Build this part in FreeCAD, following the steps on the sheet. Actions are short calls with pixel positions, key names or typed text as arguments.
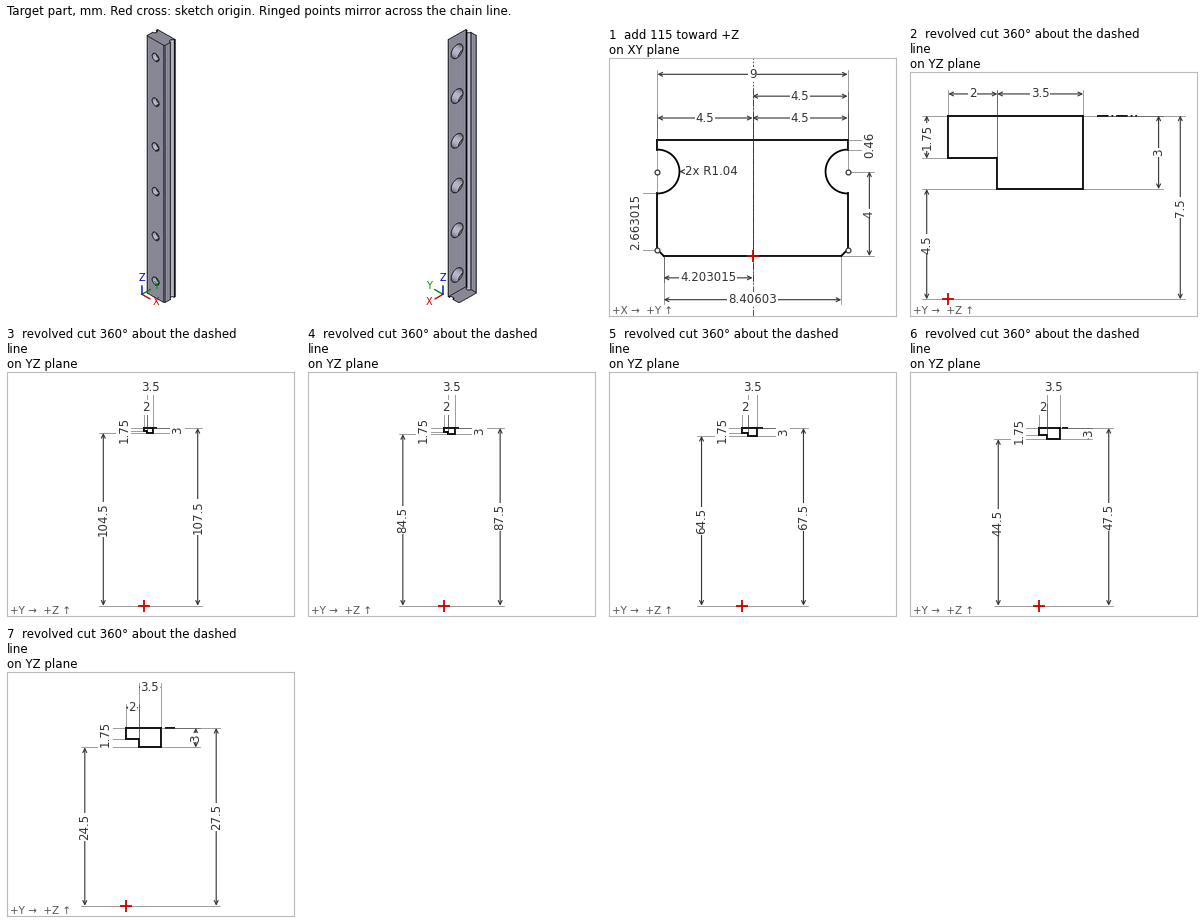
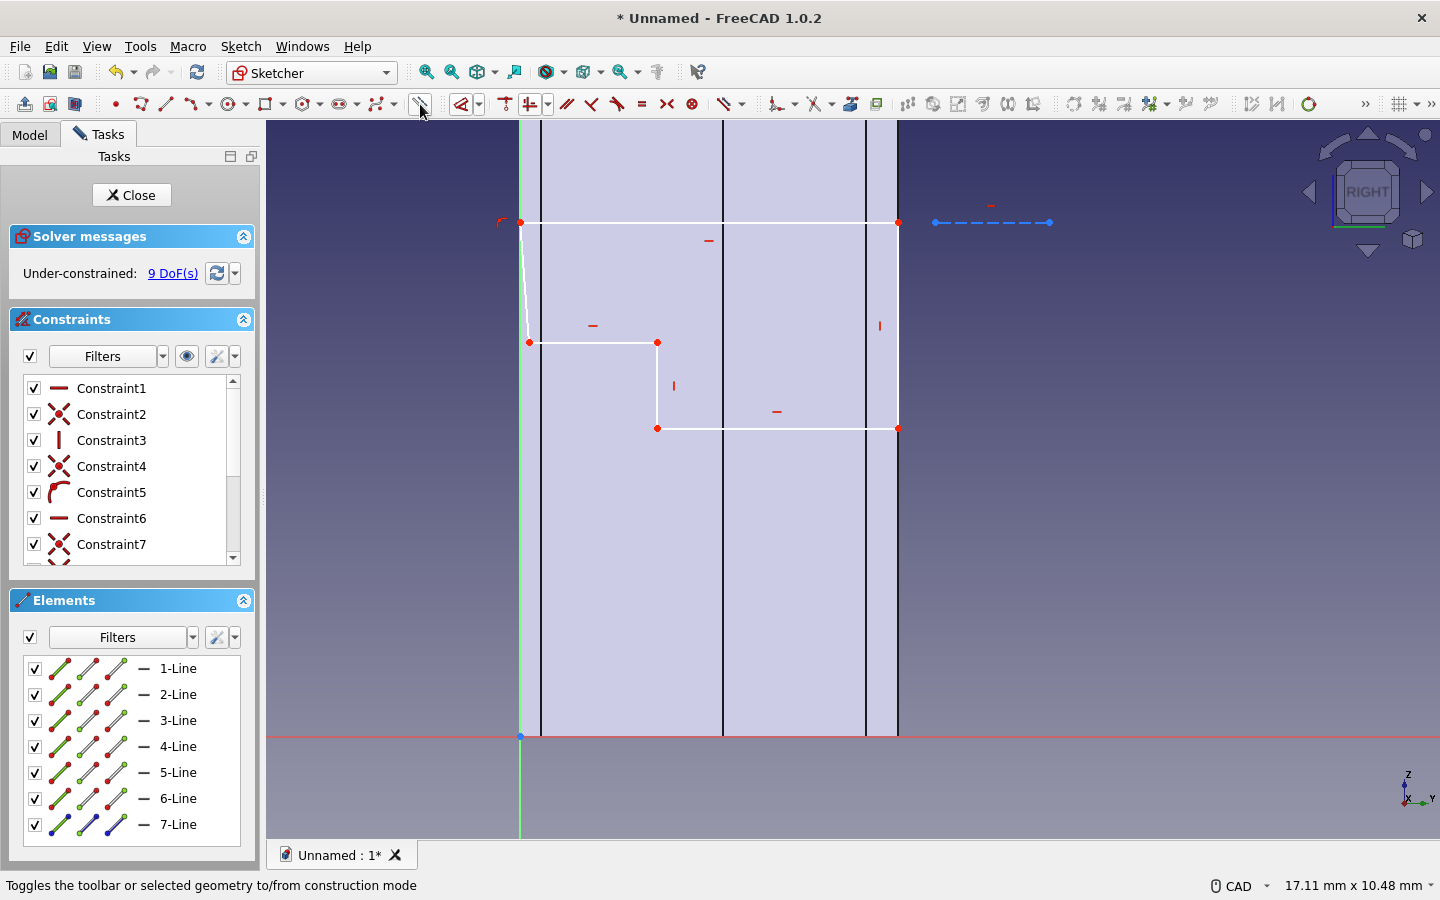
click(523, 259)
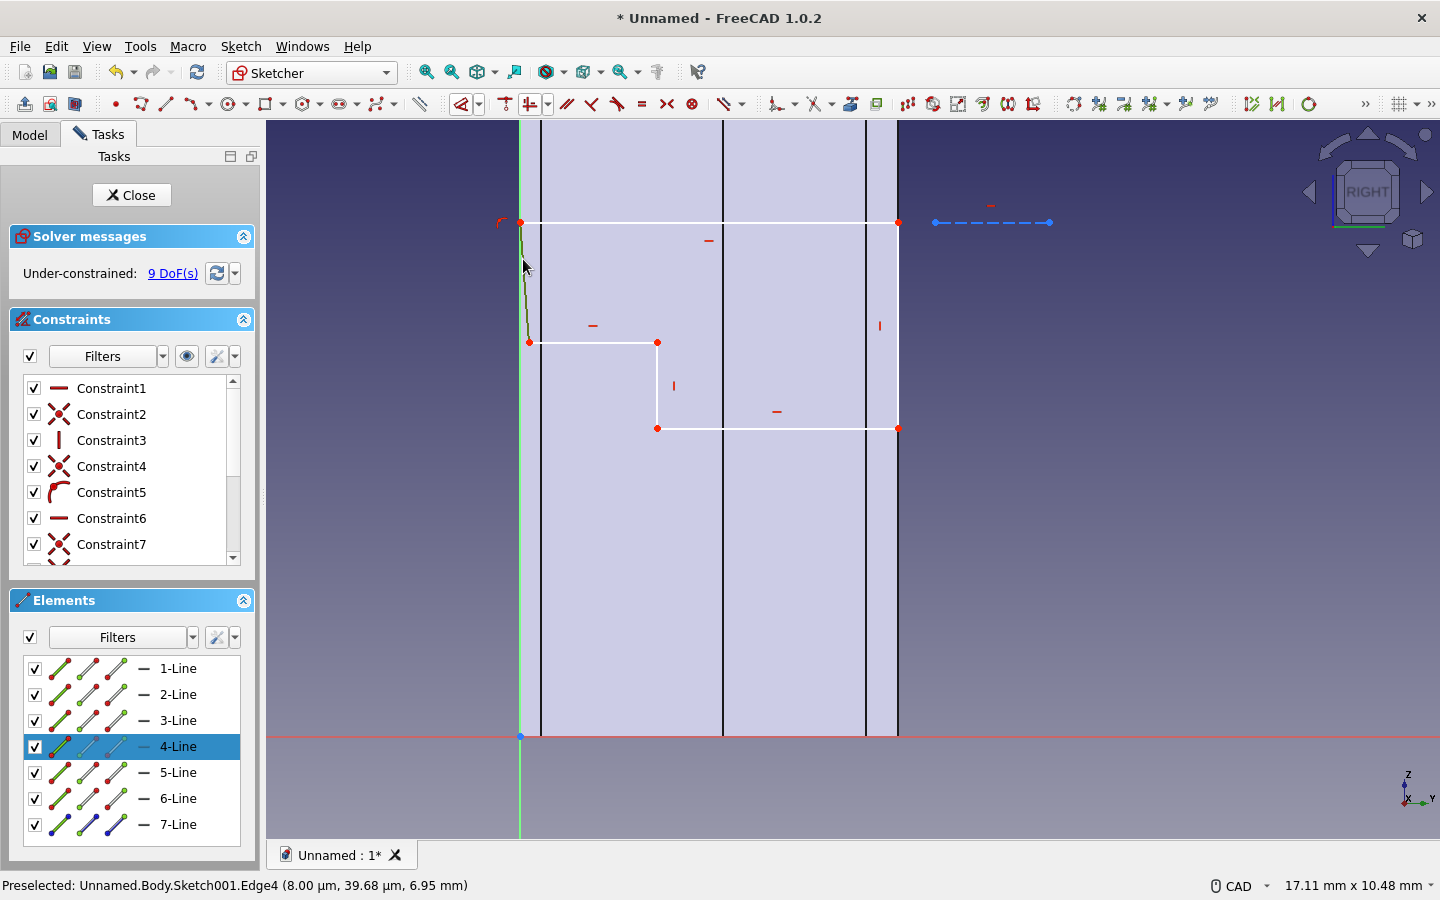
key(v)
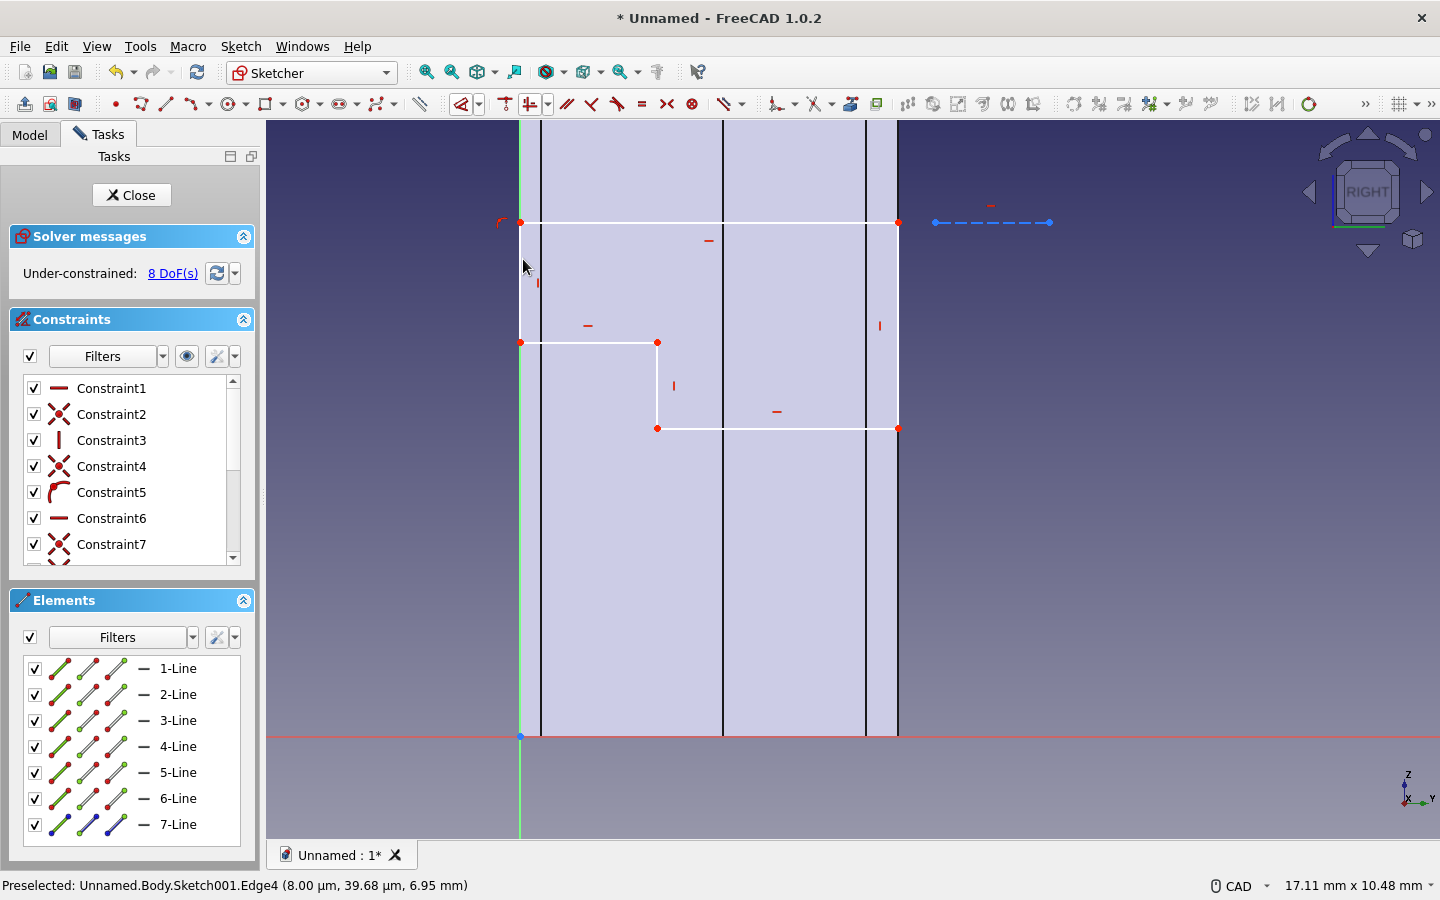
click(460, 104)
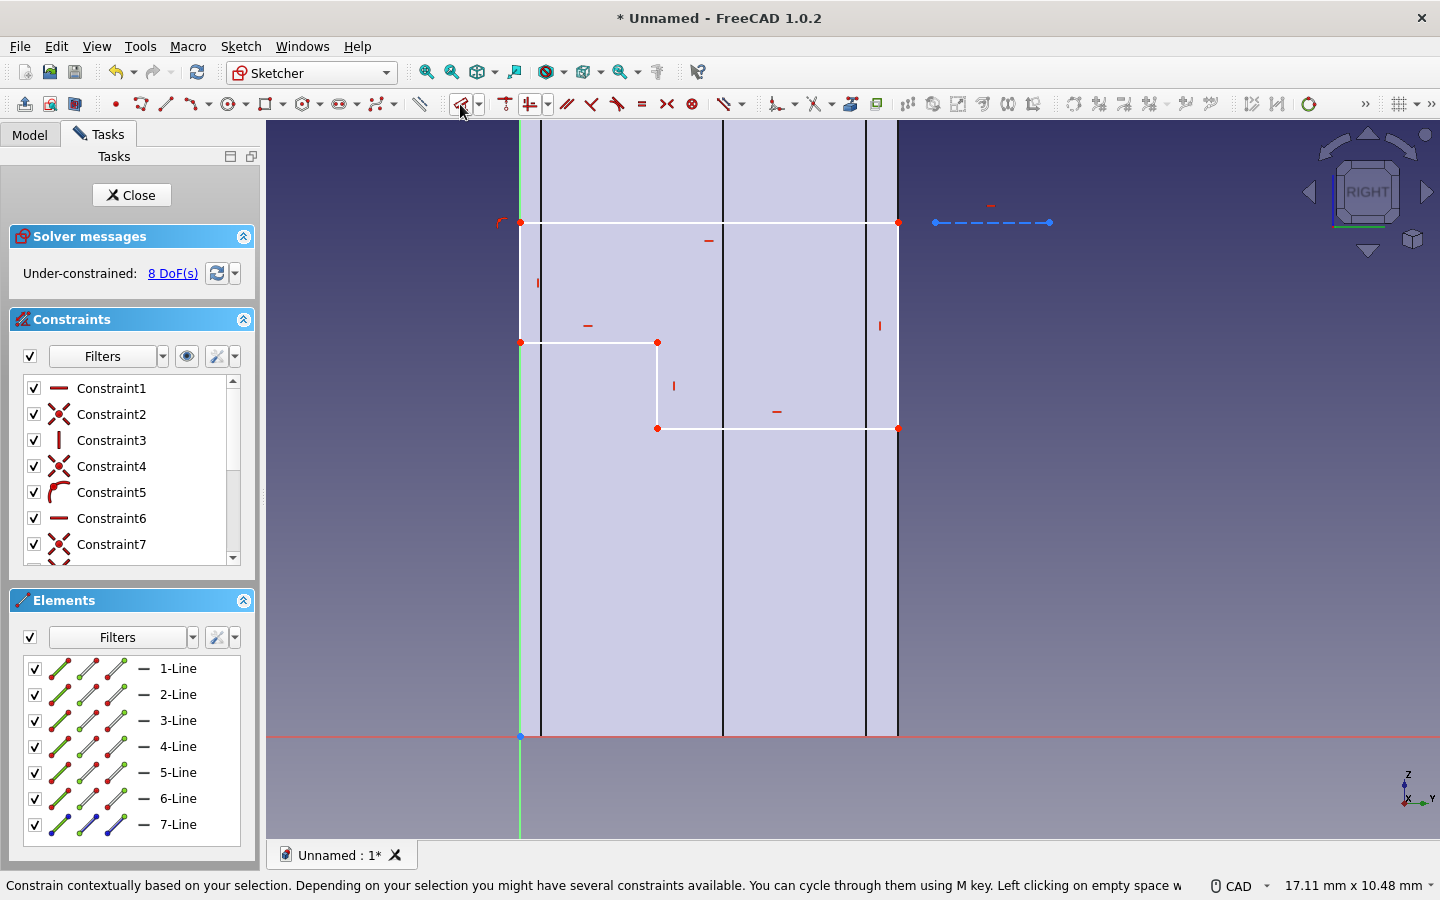
click(898, 367)
click(932, 326)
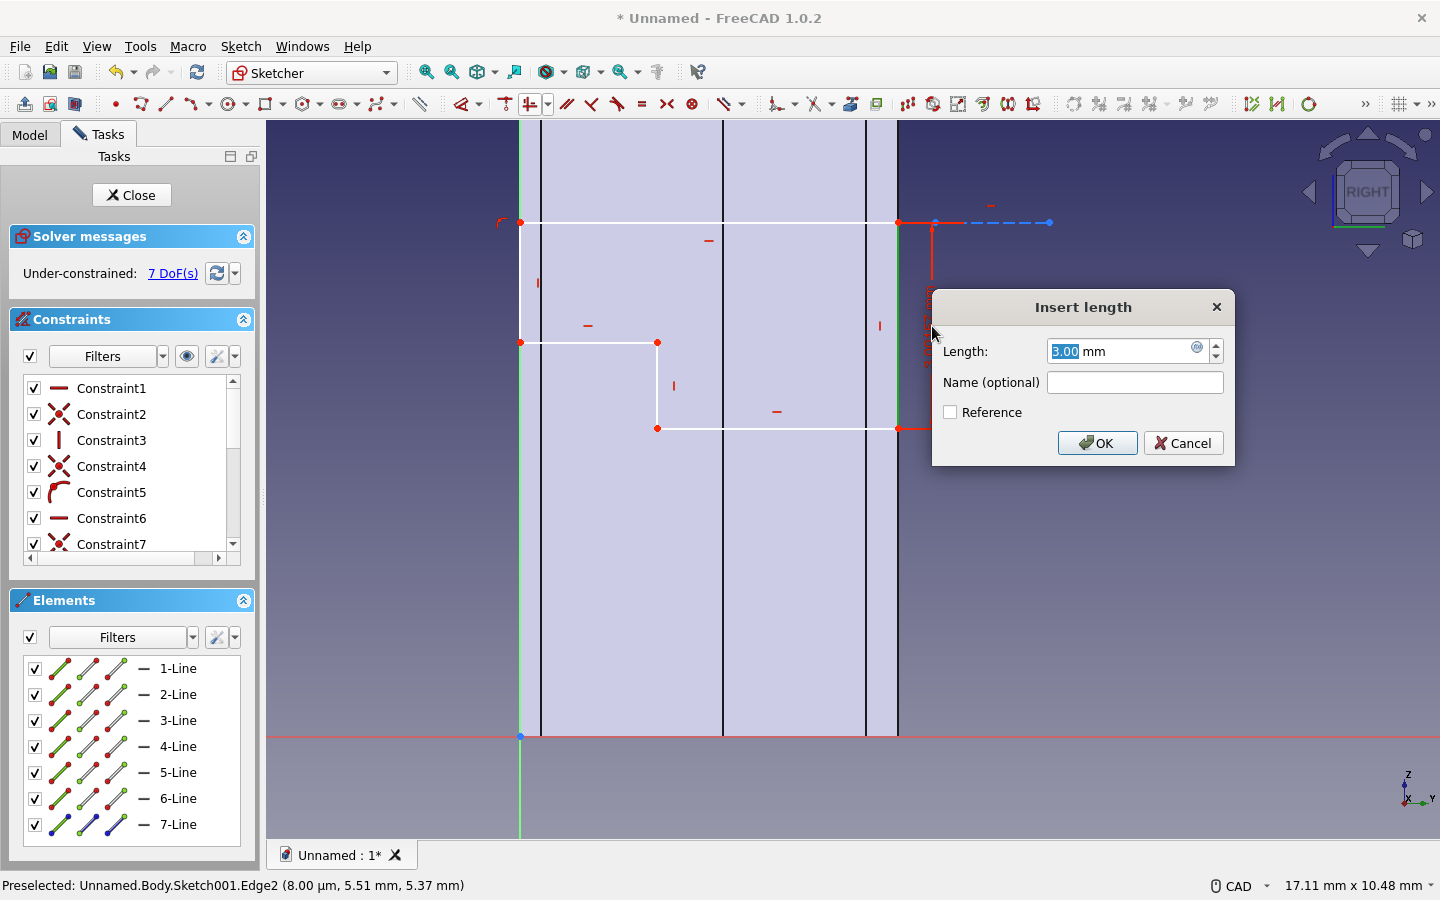
text(3)
key(Return)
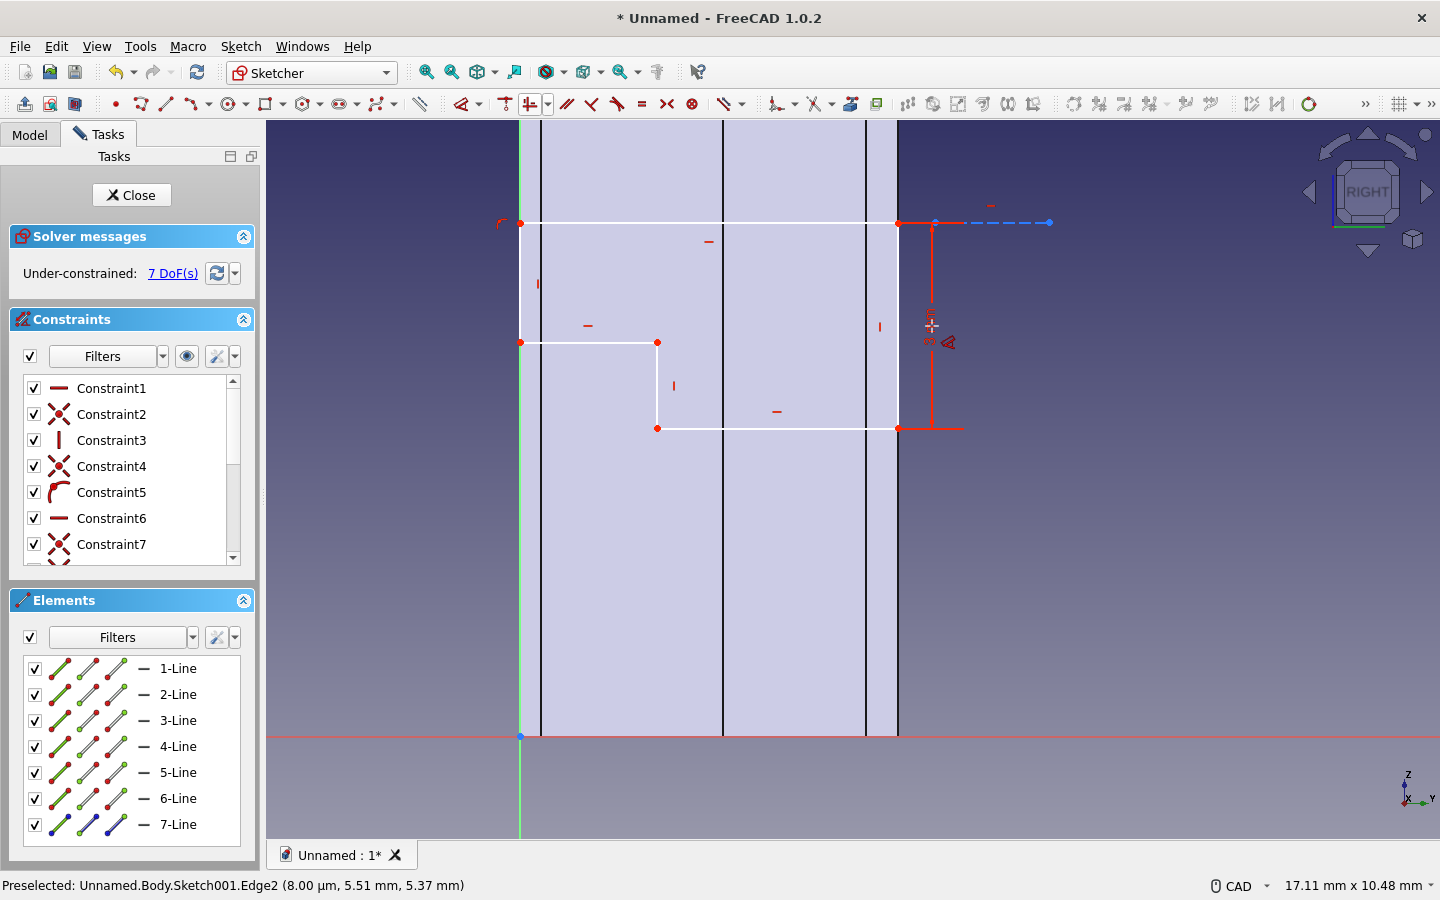
click(561, 343)
click(589, 309)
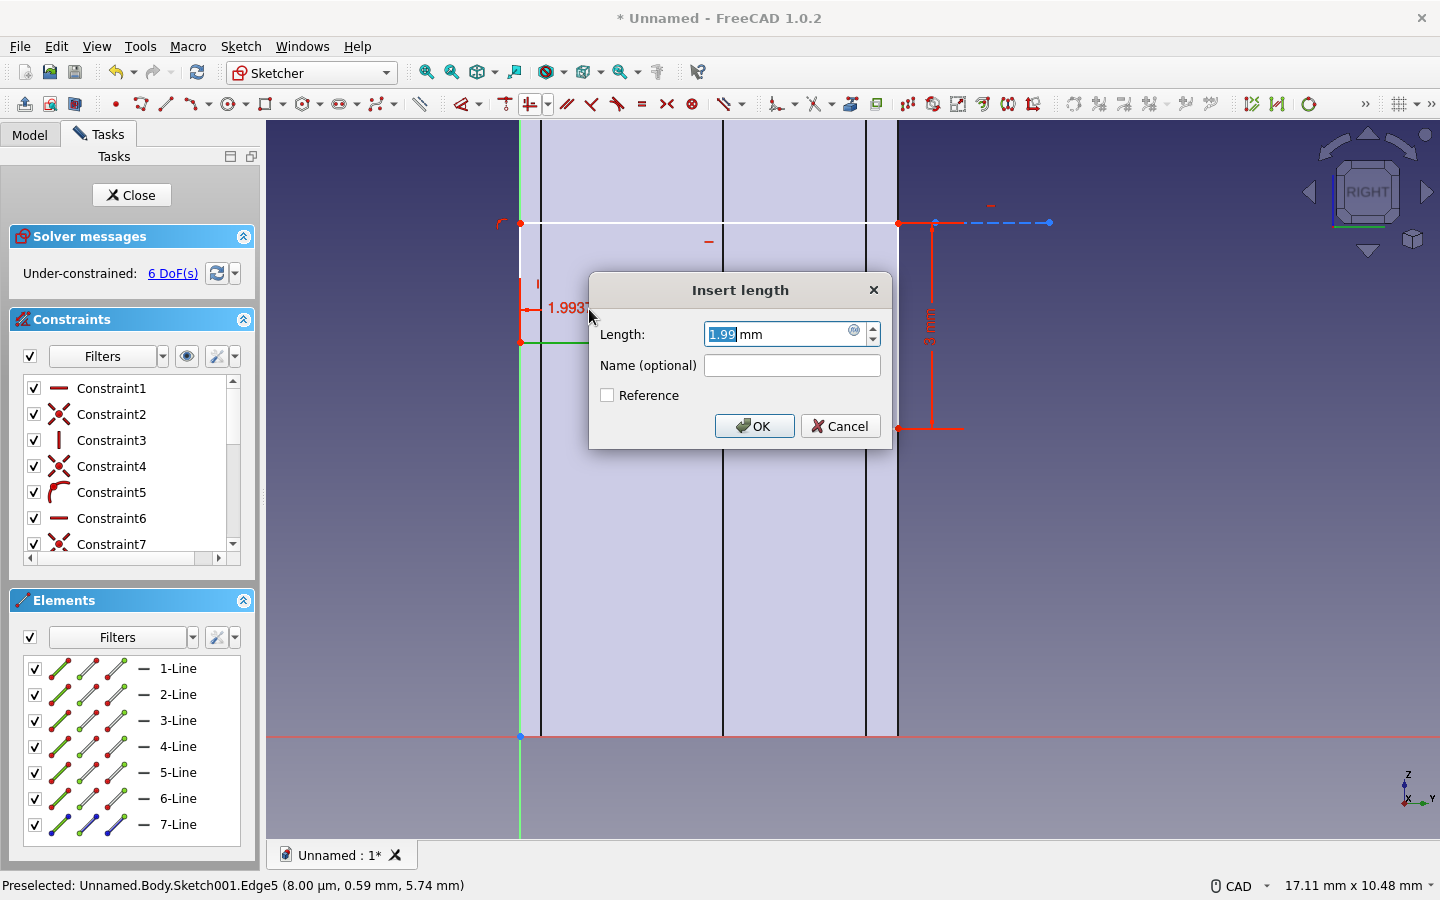
text(2)
key(Return)